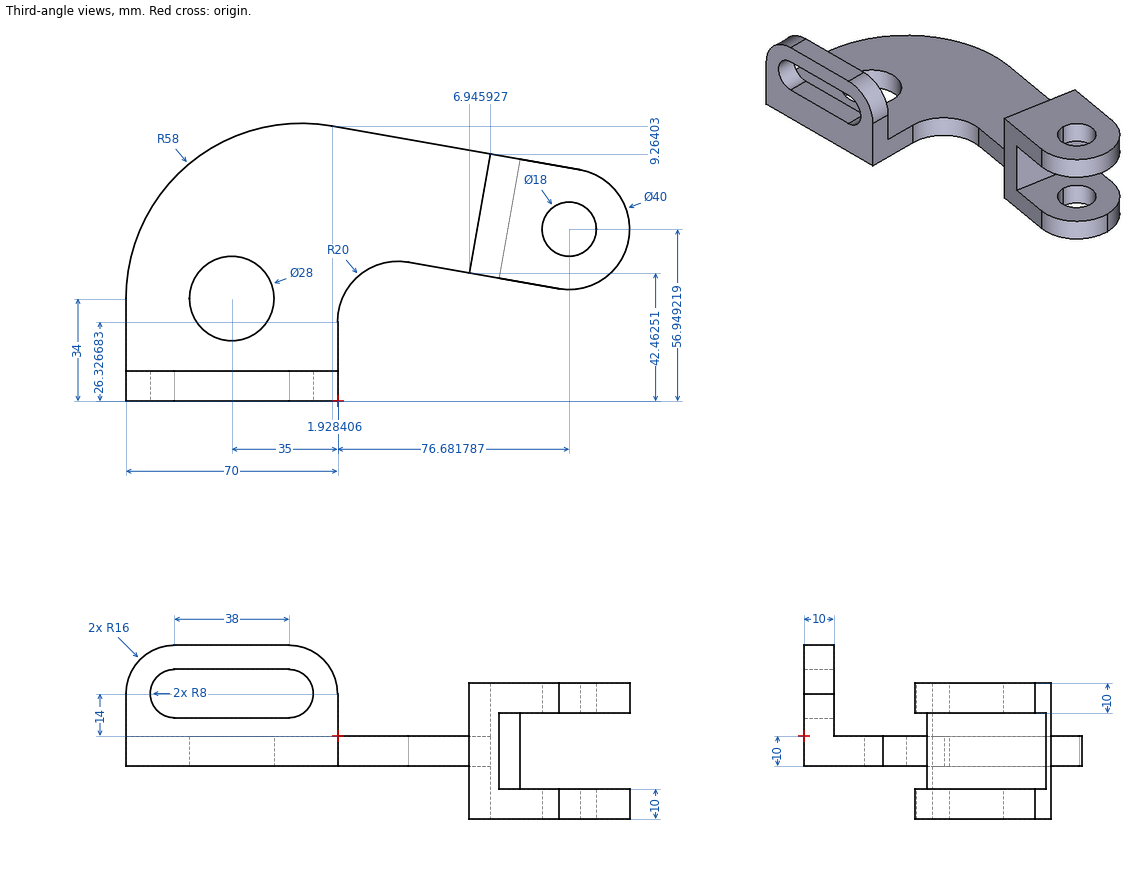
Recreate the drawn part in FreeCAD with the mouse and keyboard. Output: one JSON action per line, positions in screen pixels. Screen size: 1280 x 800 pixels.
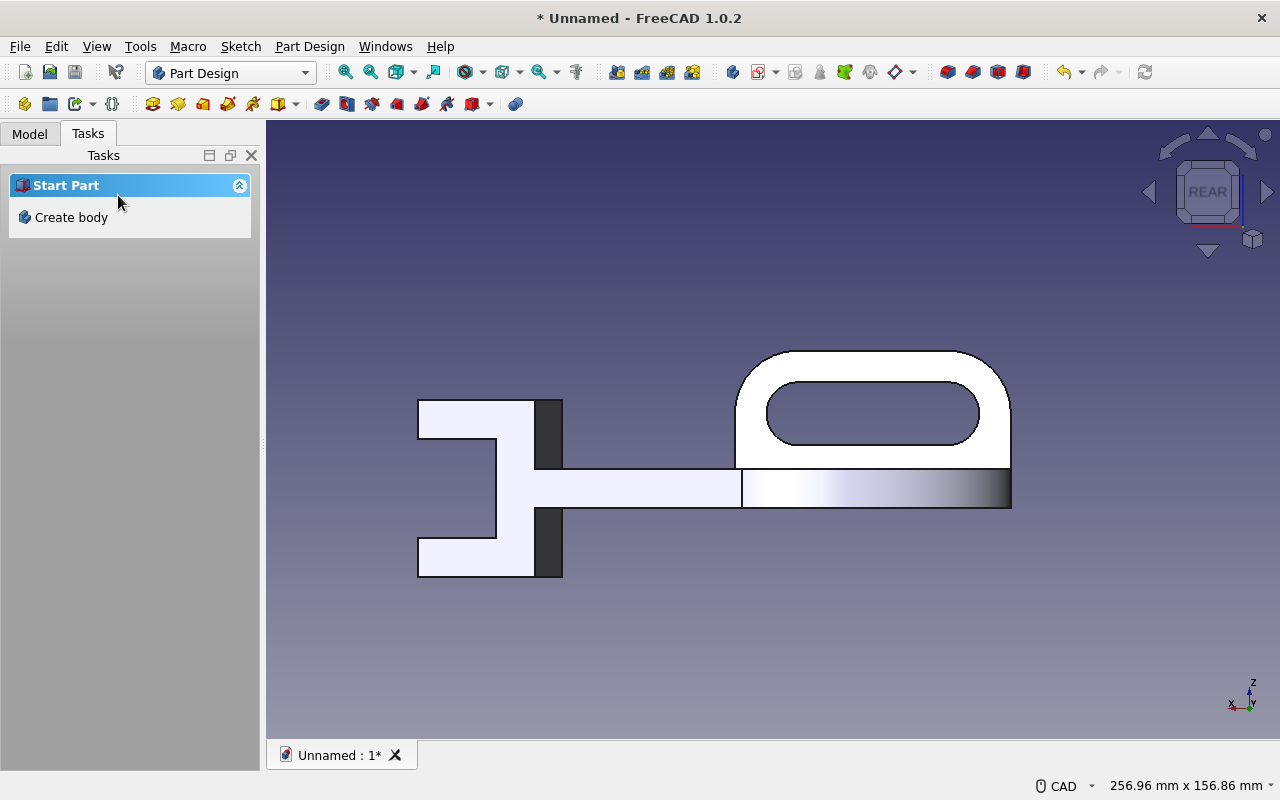
{"action": "key", "text": "0"}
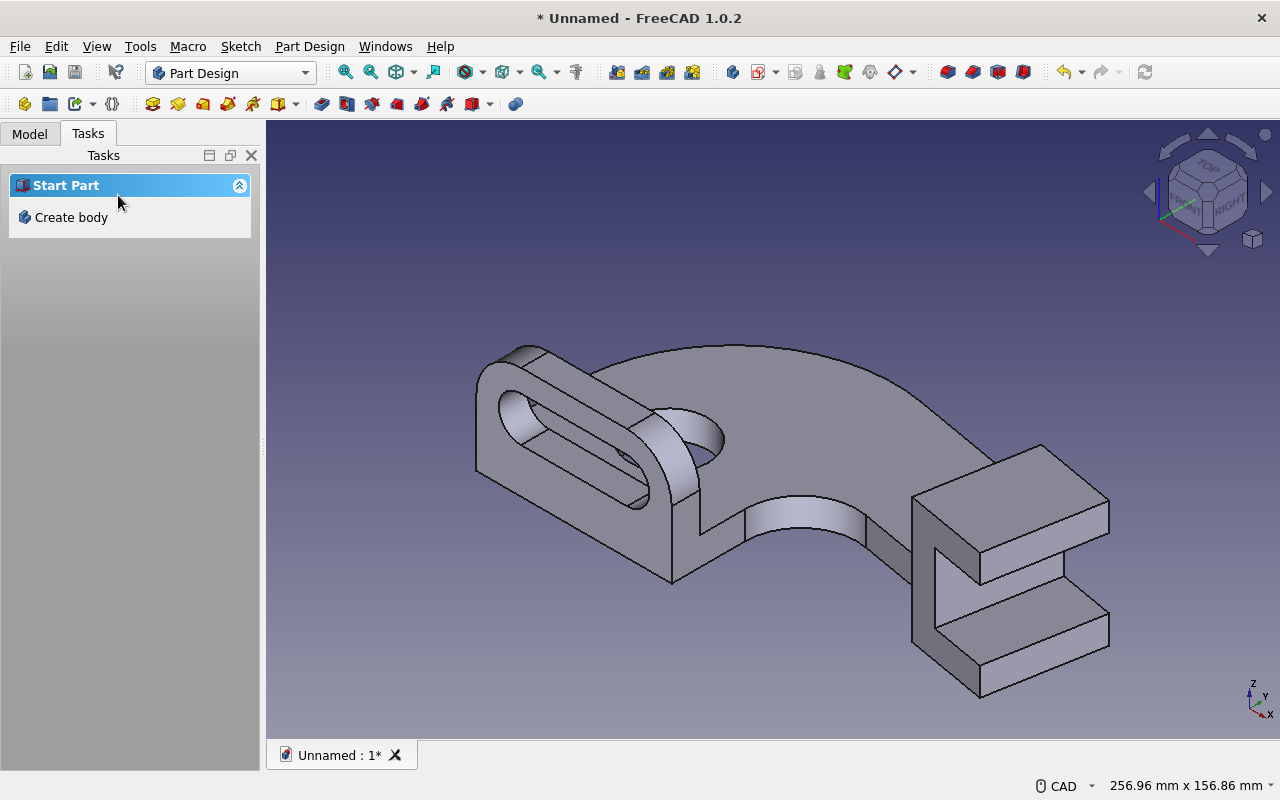
{"action": "left_click", "coordinate": [346, 72]}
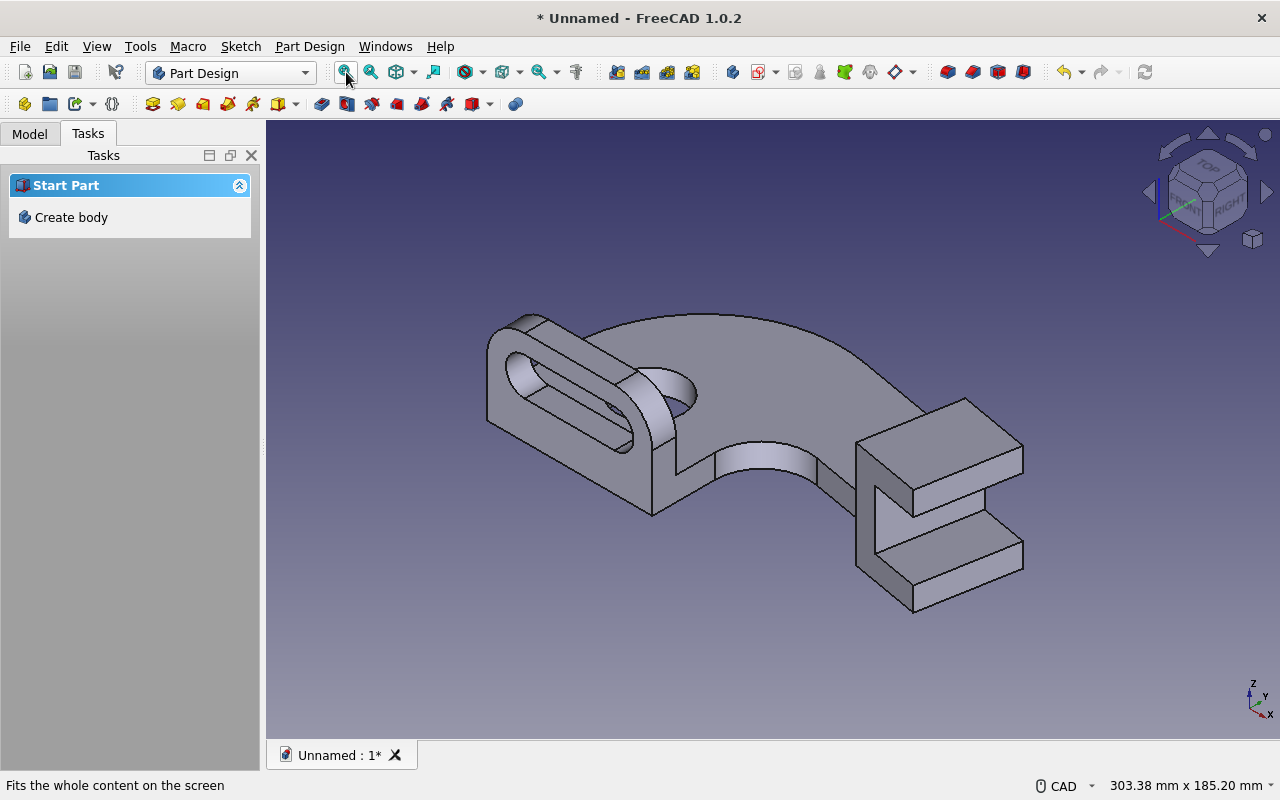
{"action": "left_click", "coordinate": [939, 443]}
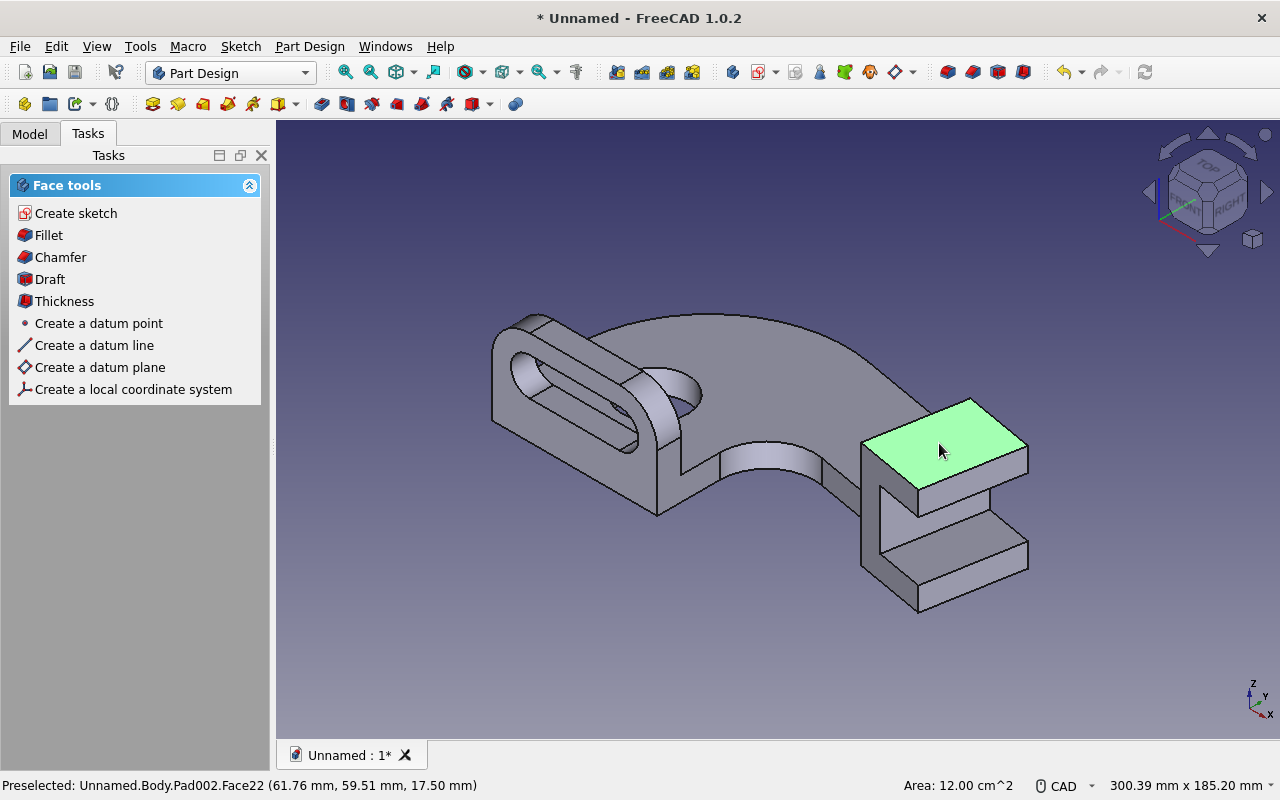
{"action": "left_click", "coordinate": [758, 72]}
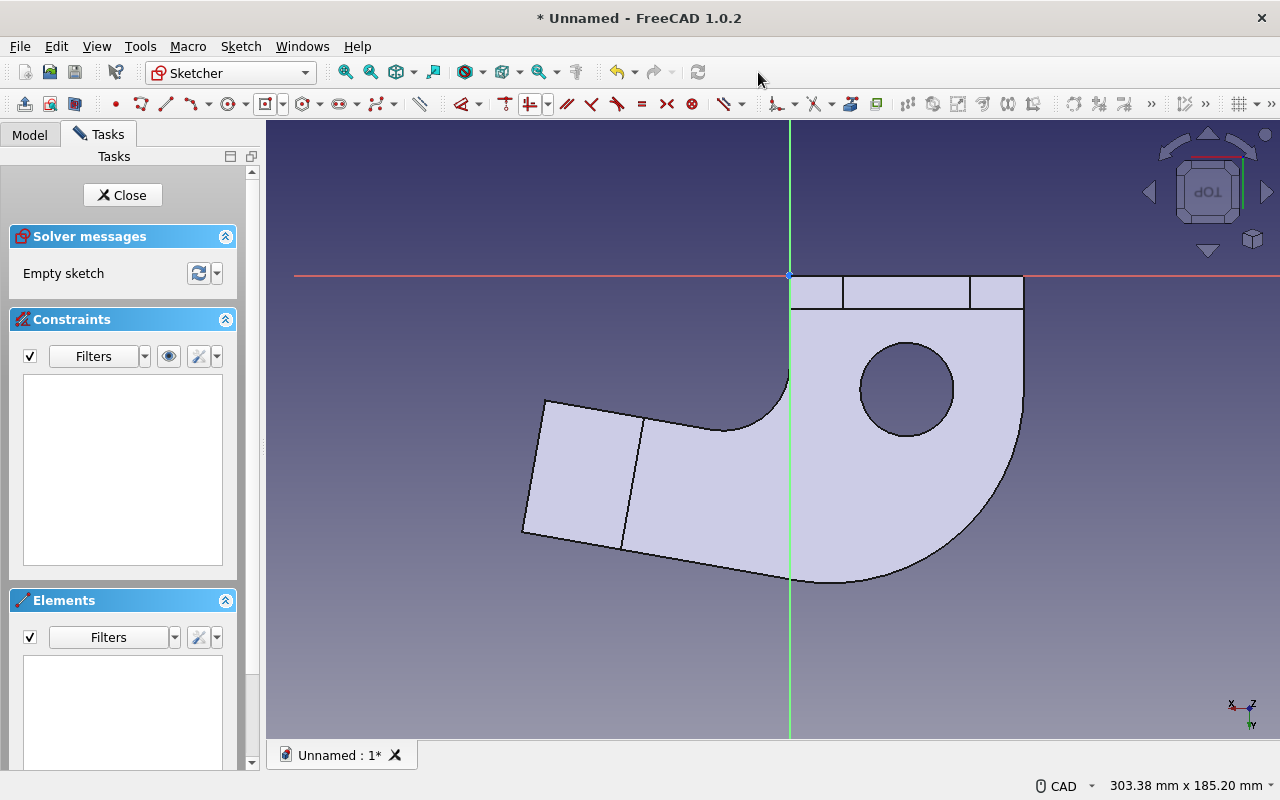
{"action": "scroll", "coordinate": [474, 354], "scroll_direction": "up", "scroll_amount": 2}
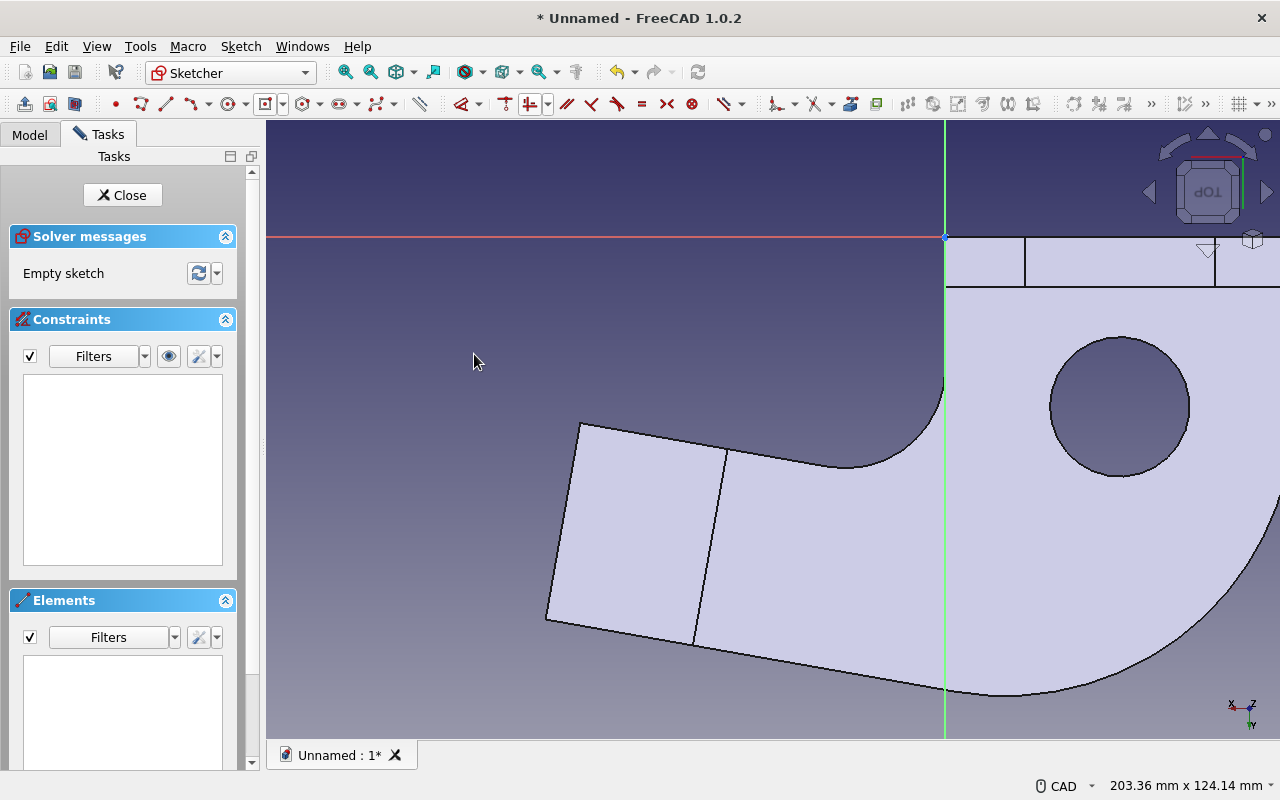
{"action": "left_click", "coordinate": [228, 104]}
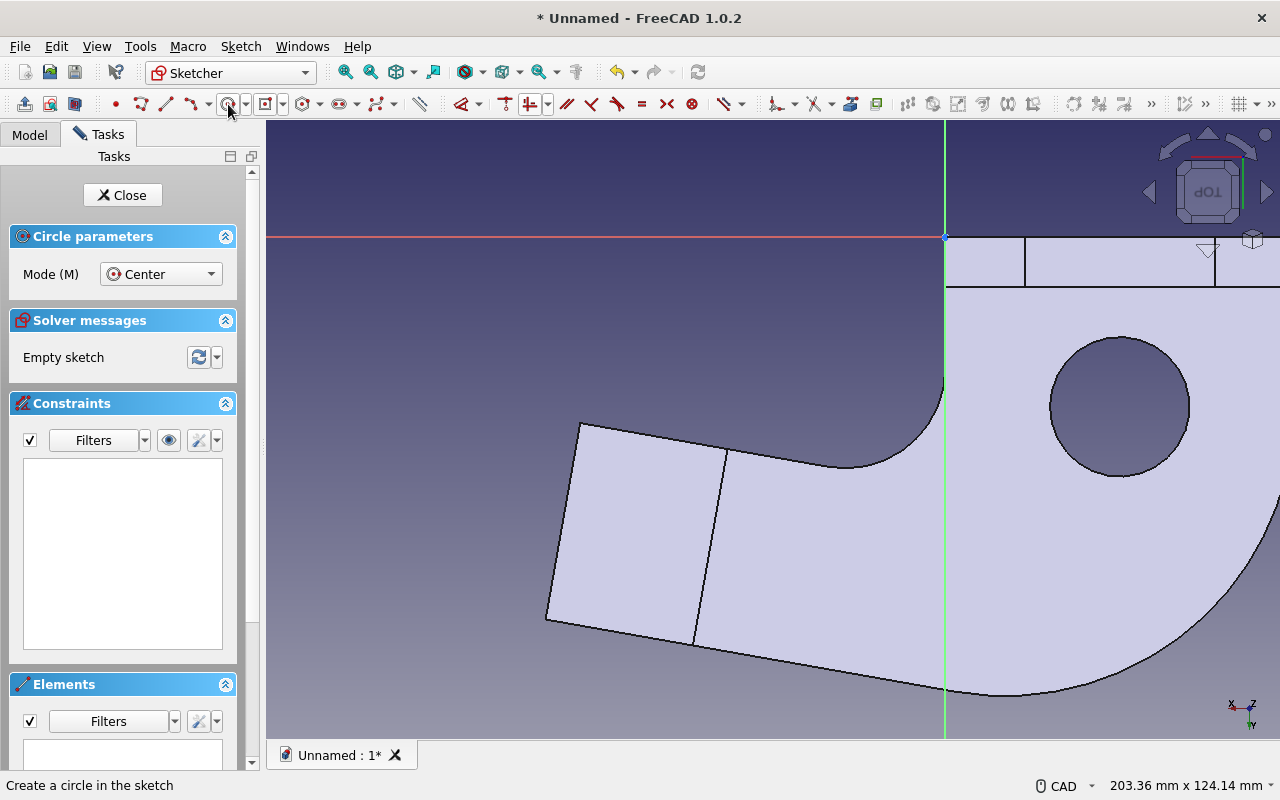
{"action": "left_click", "coordinate": [563, 521]}
{"action": "left_click", "coordinate": [633, 451]}
{"action": "key", "text": "Escape"}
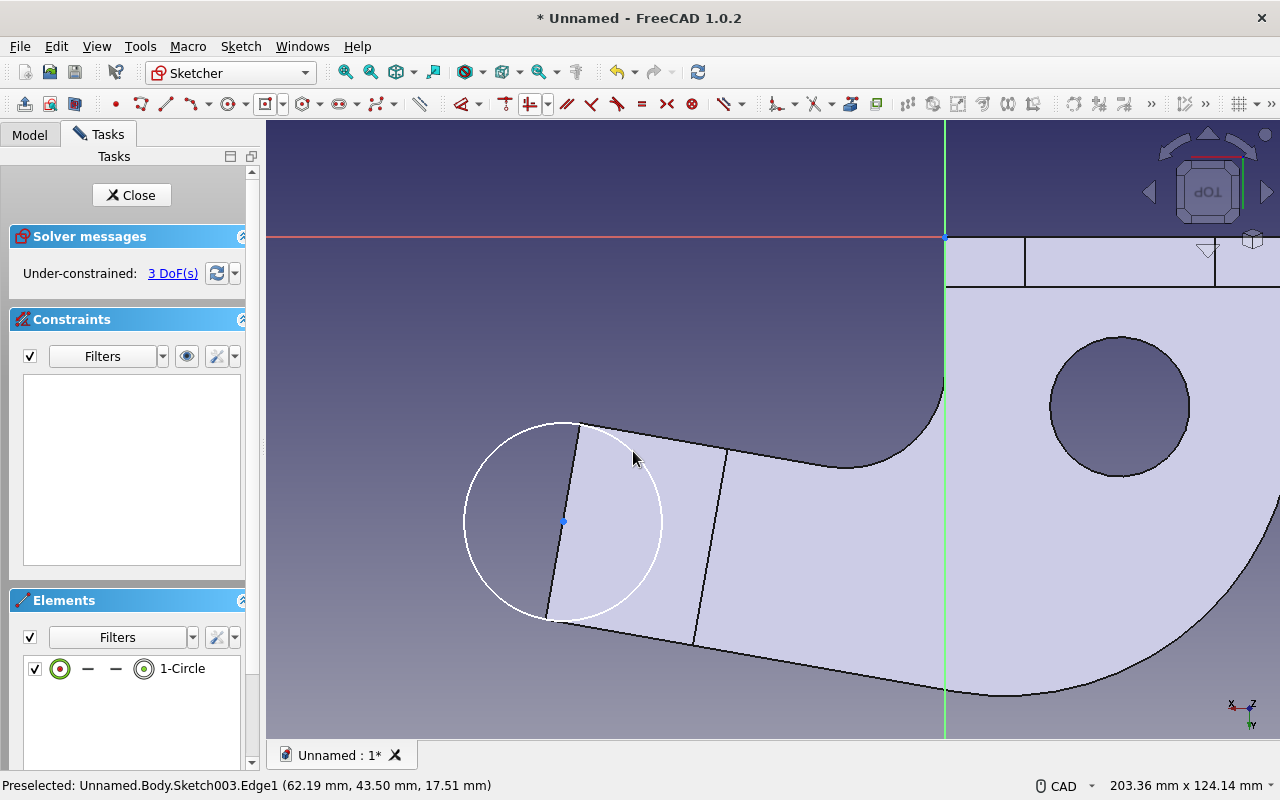
{"action": "left_click", "coordinate": [460, 104]}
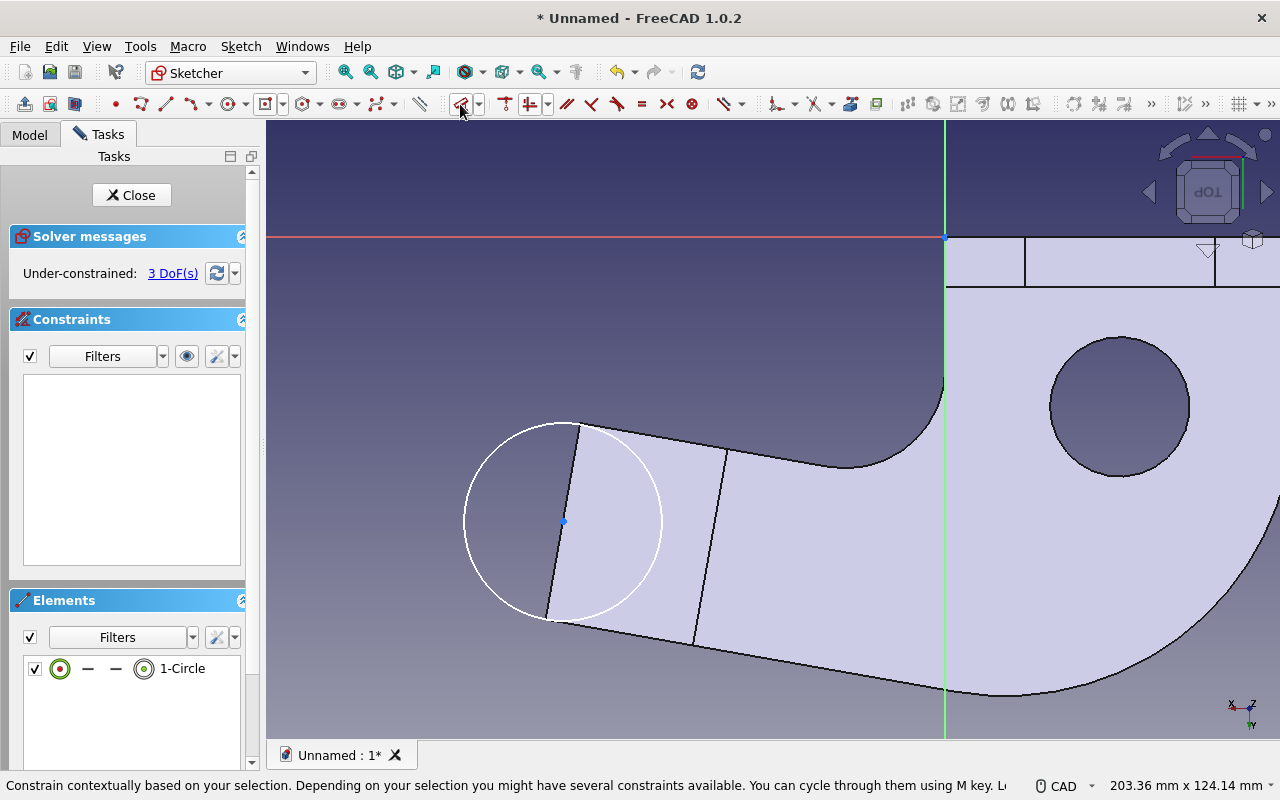
{"action": "left_click", "coordinate": [633, 452]}
{"action": "left_click", "coordinate": [656, 429]}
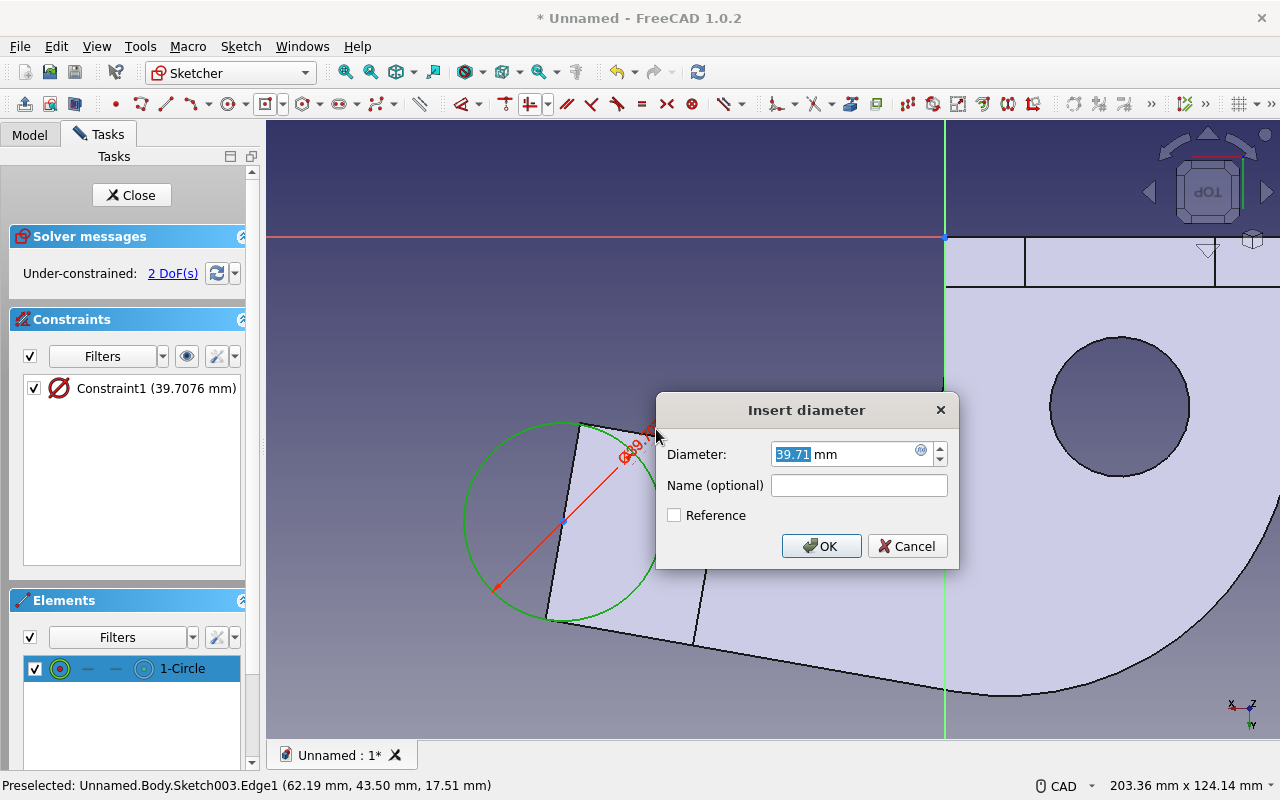
{"action": "type", "text": "40"}
{"action": "key", "text": "Return"}